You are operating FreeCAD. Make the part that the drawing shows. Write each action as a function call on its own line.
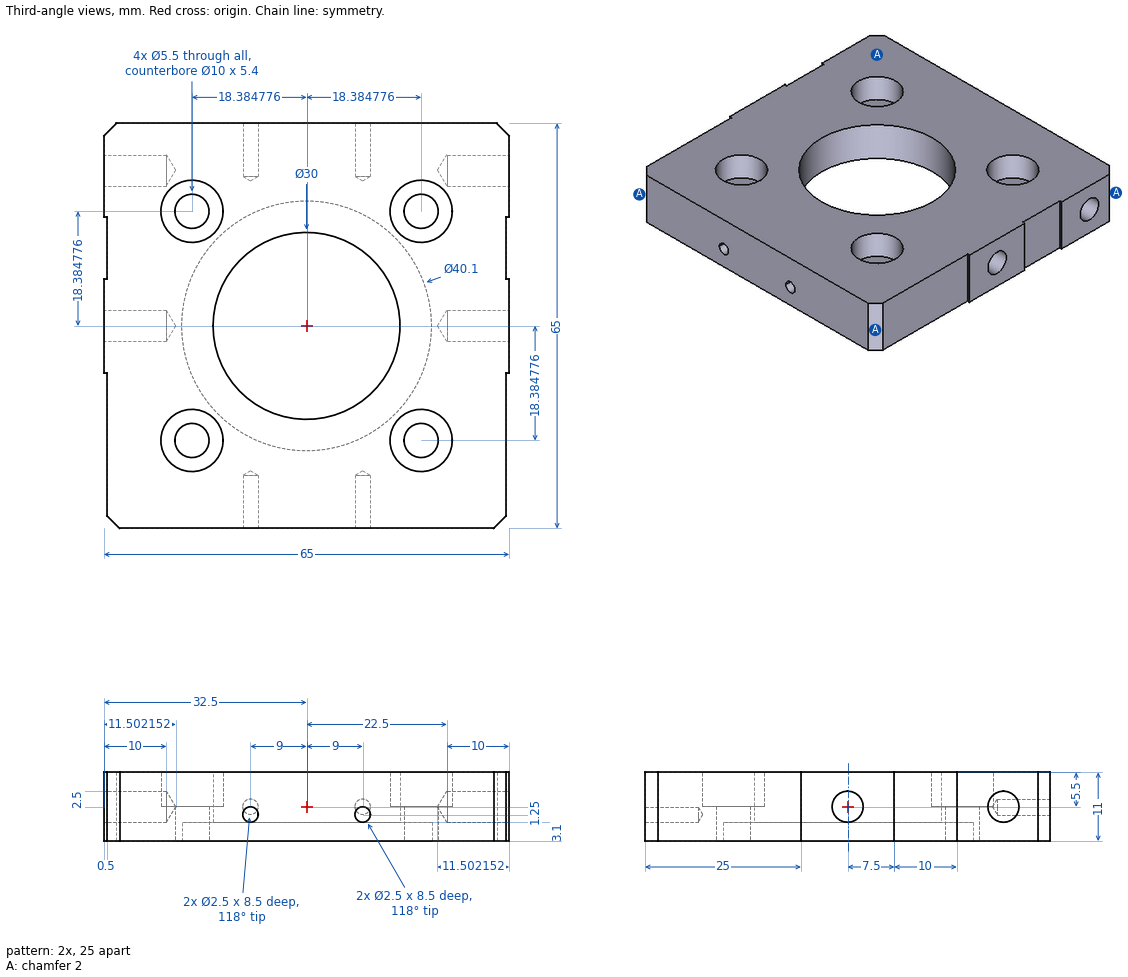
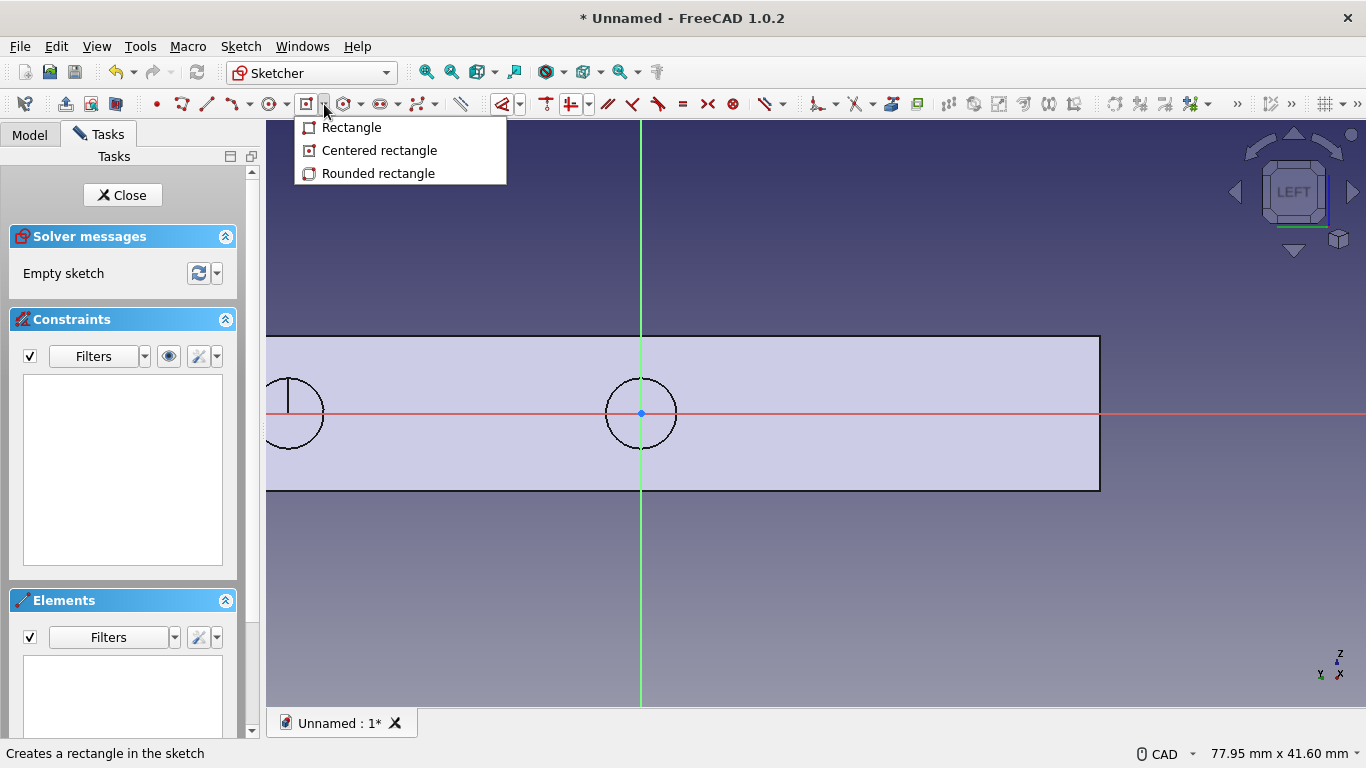
click(400, 128)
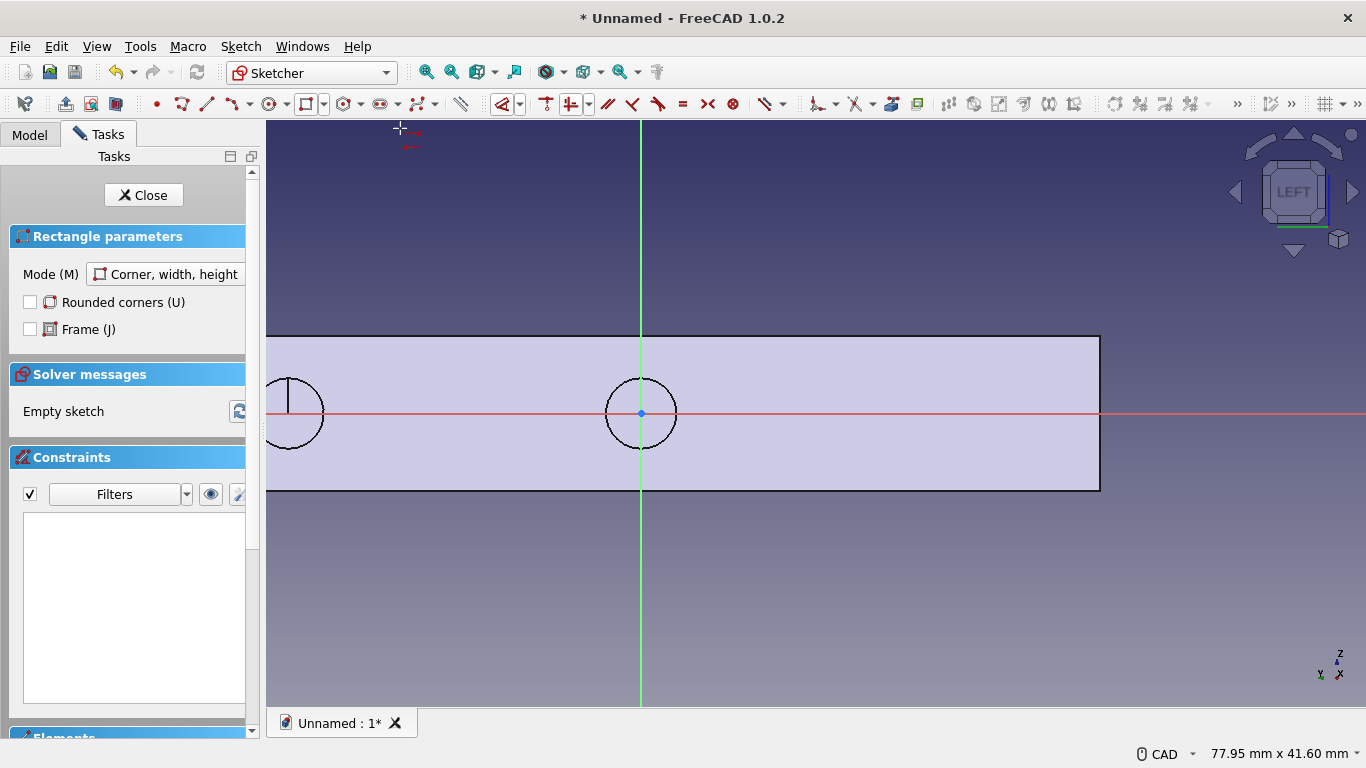
click(394, 336)
click(535, 491)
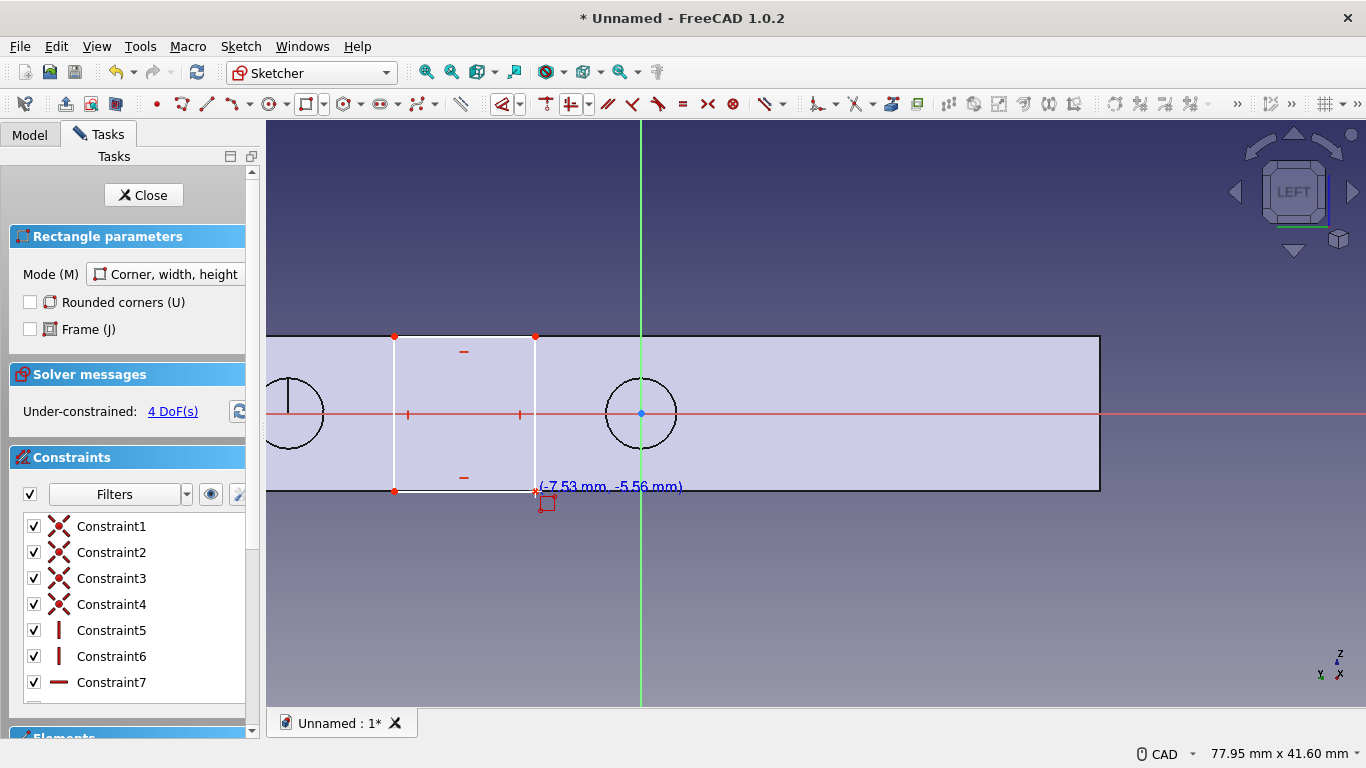
click(747, 336)
click(1100, 491)
key(Escape)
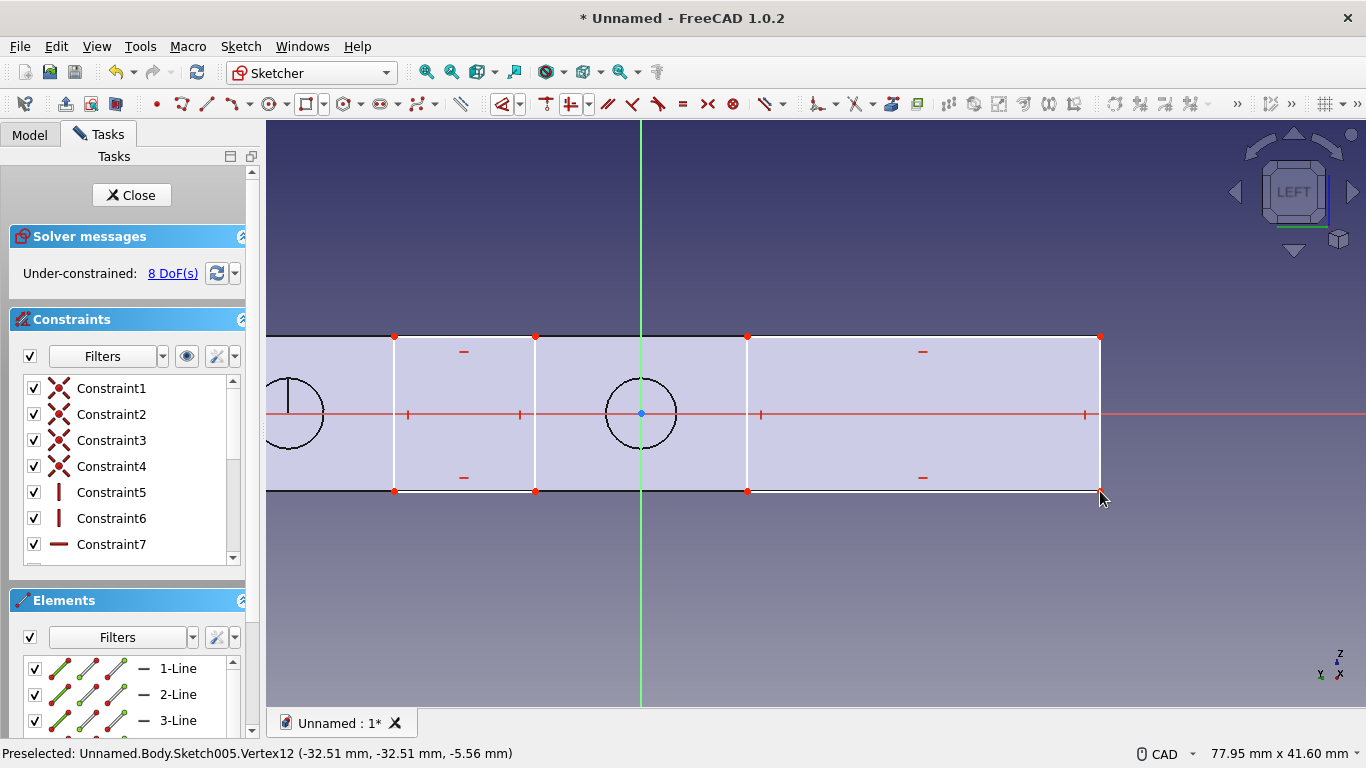
click(535, 337)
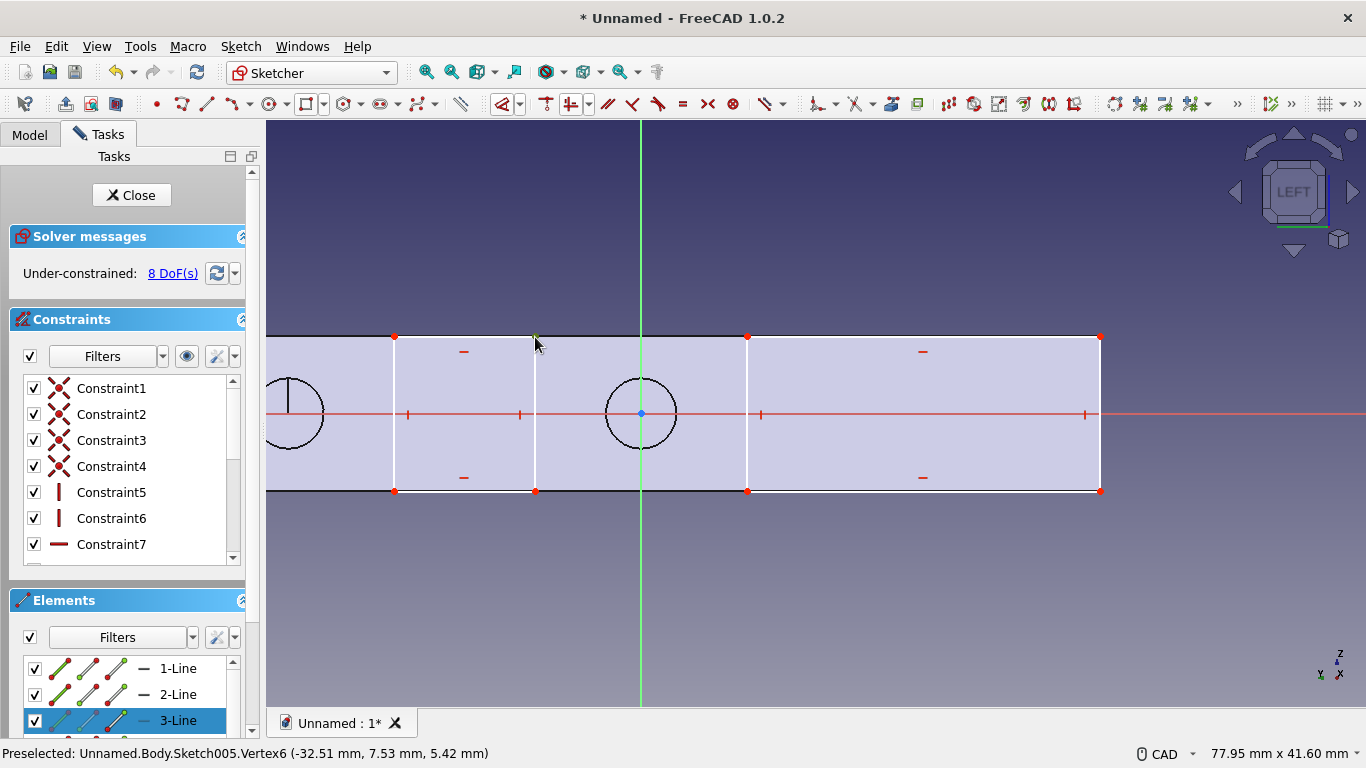
click(747, 337)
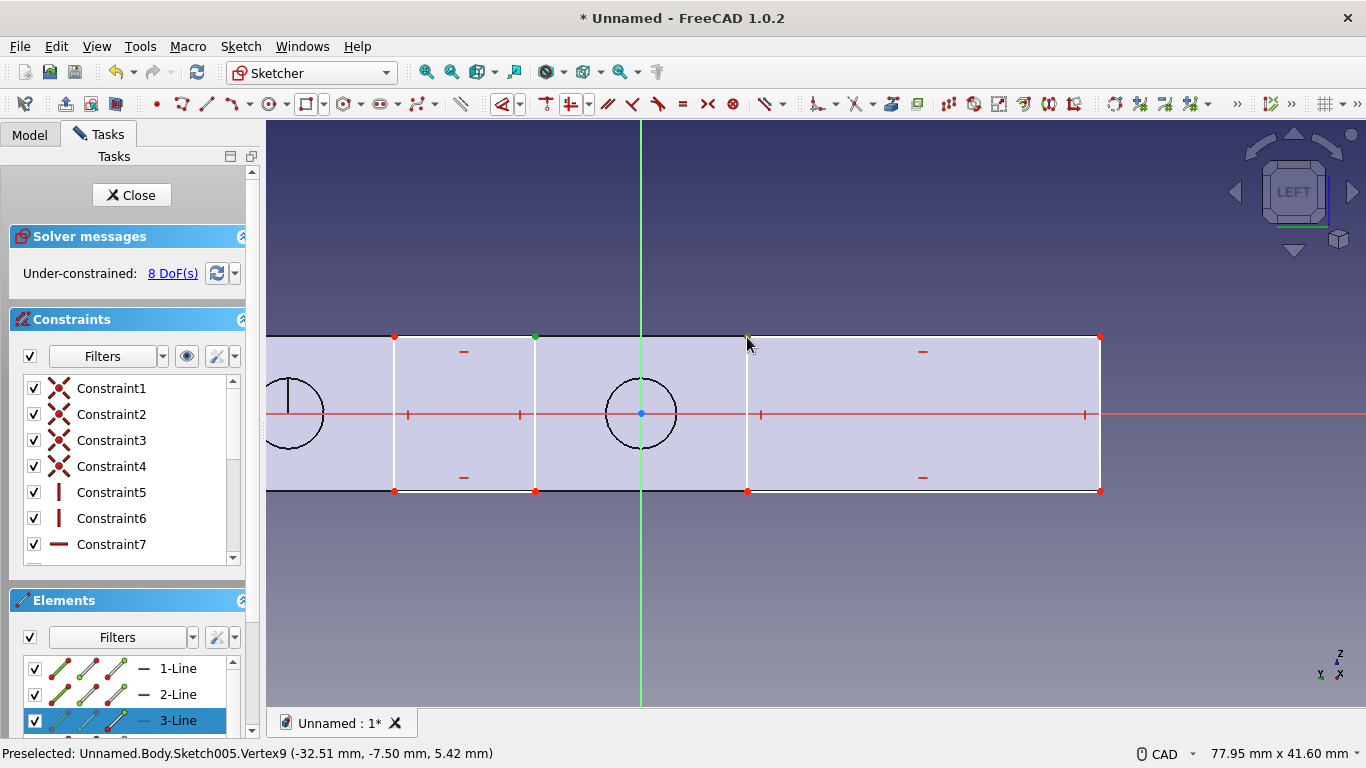
click(641, 641)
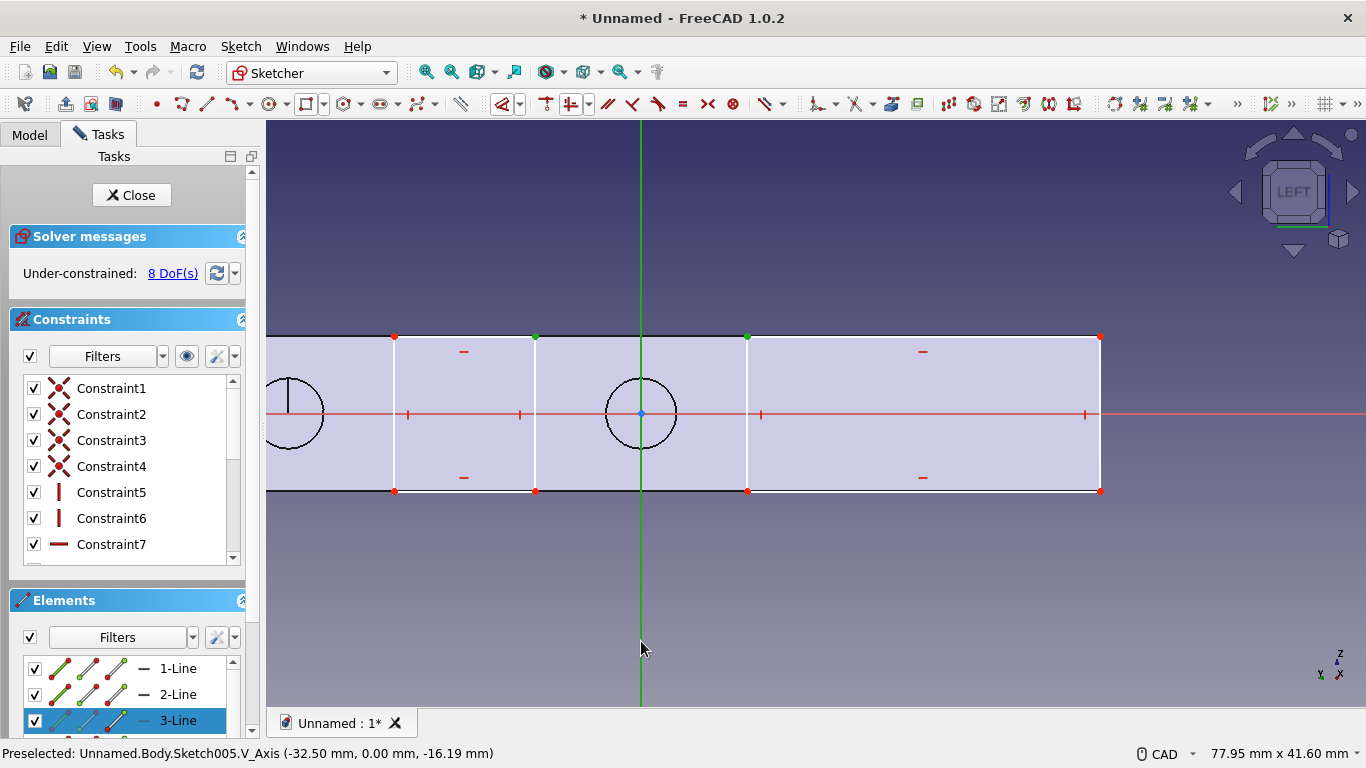
click(708, 104)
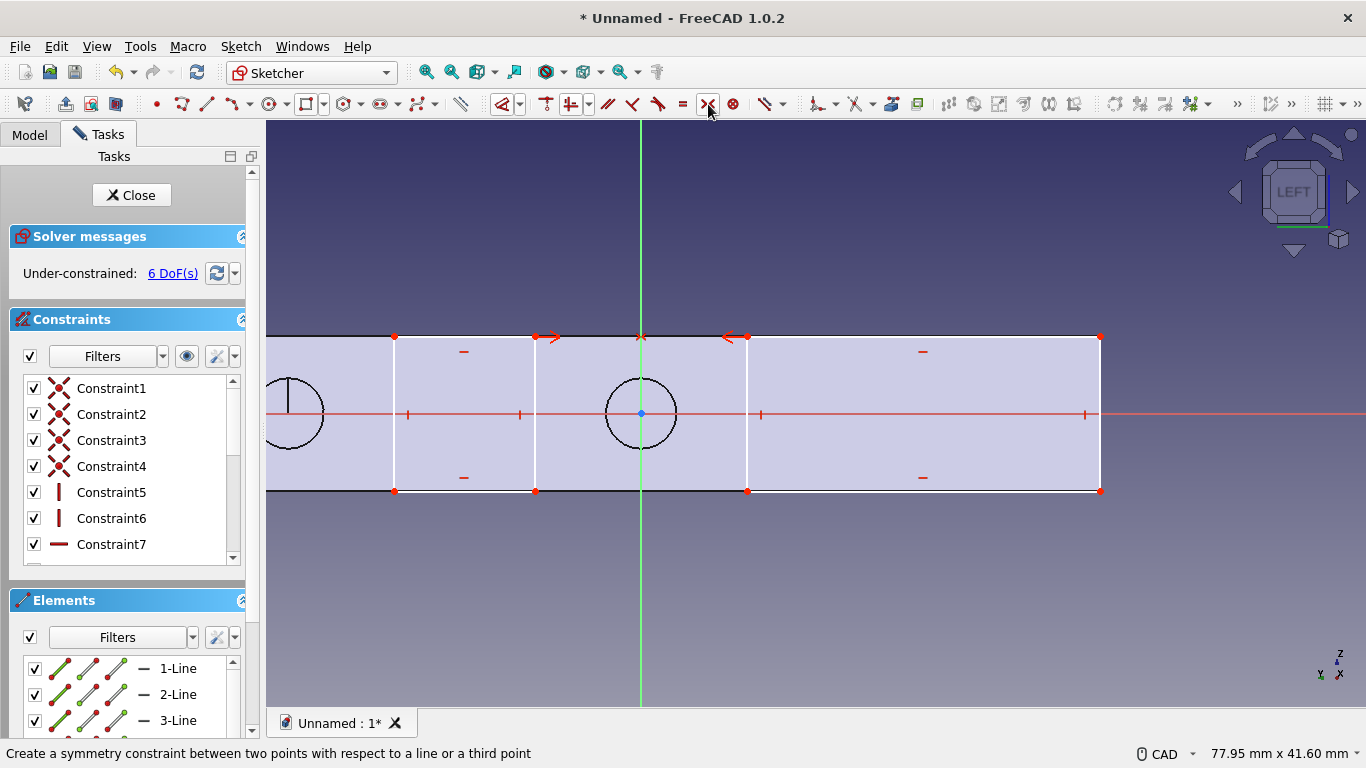
click(394, 383)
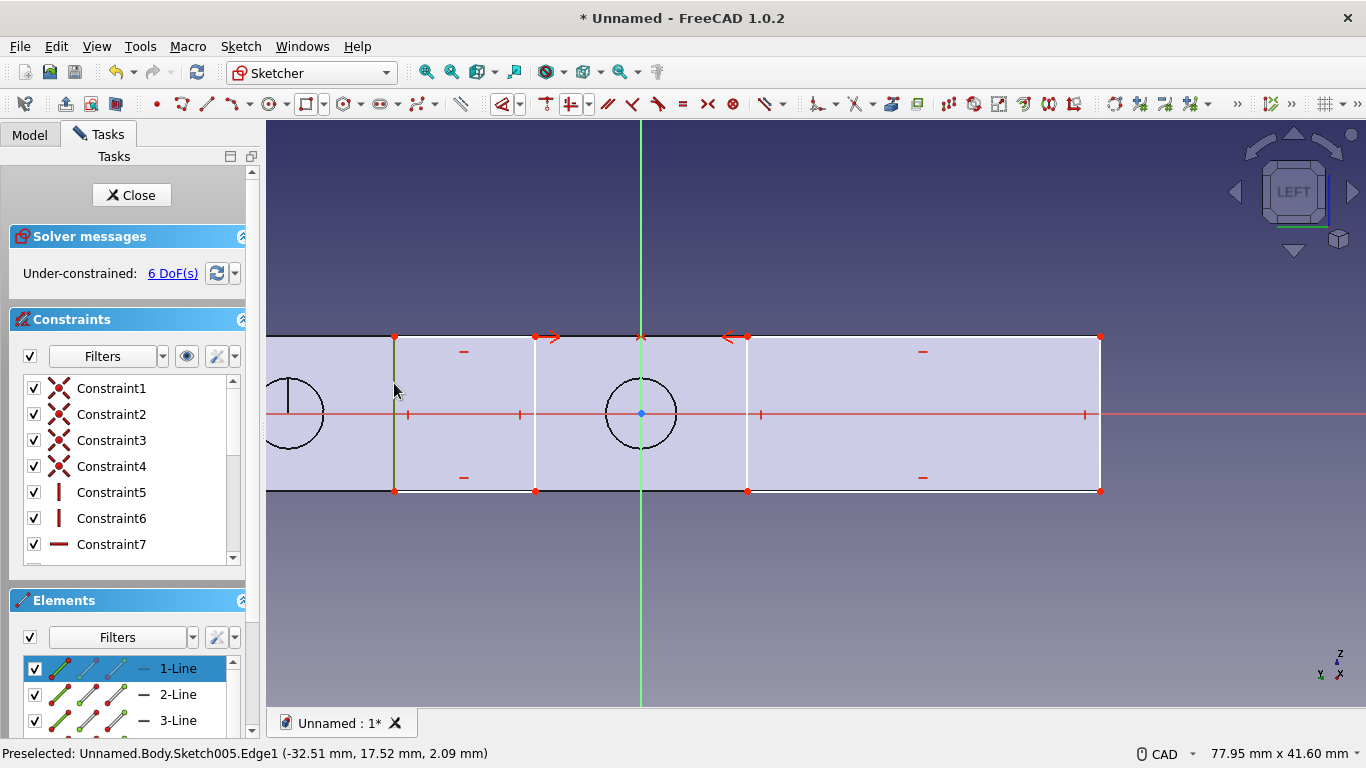
key(i)